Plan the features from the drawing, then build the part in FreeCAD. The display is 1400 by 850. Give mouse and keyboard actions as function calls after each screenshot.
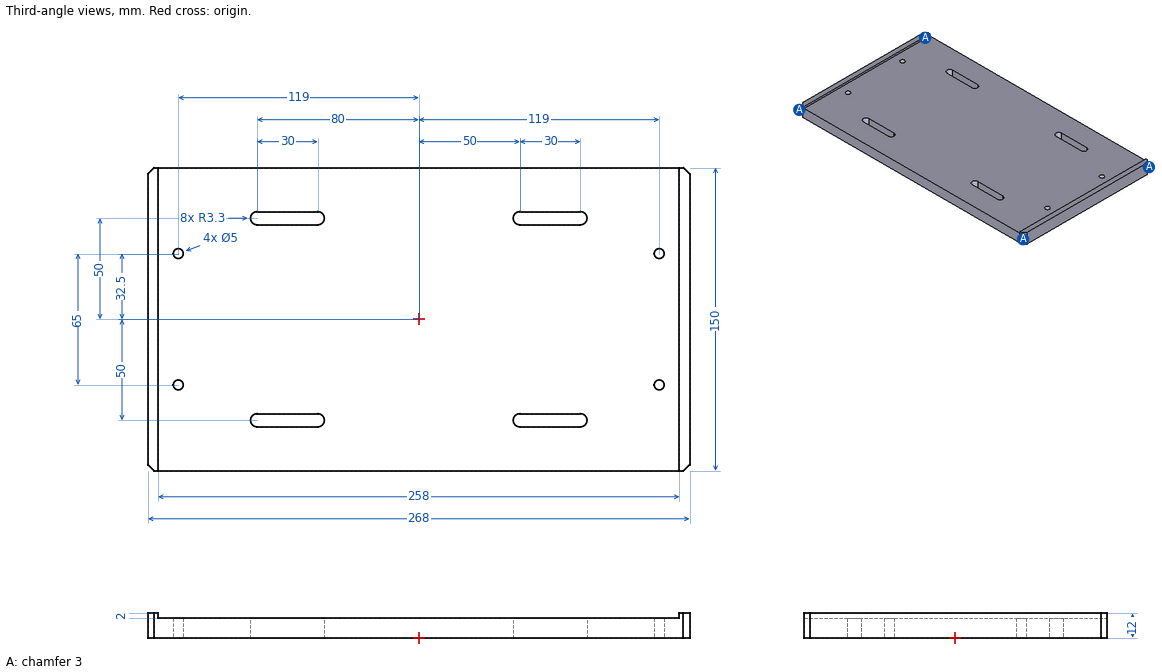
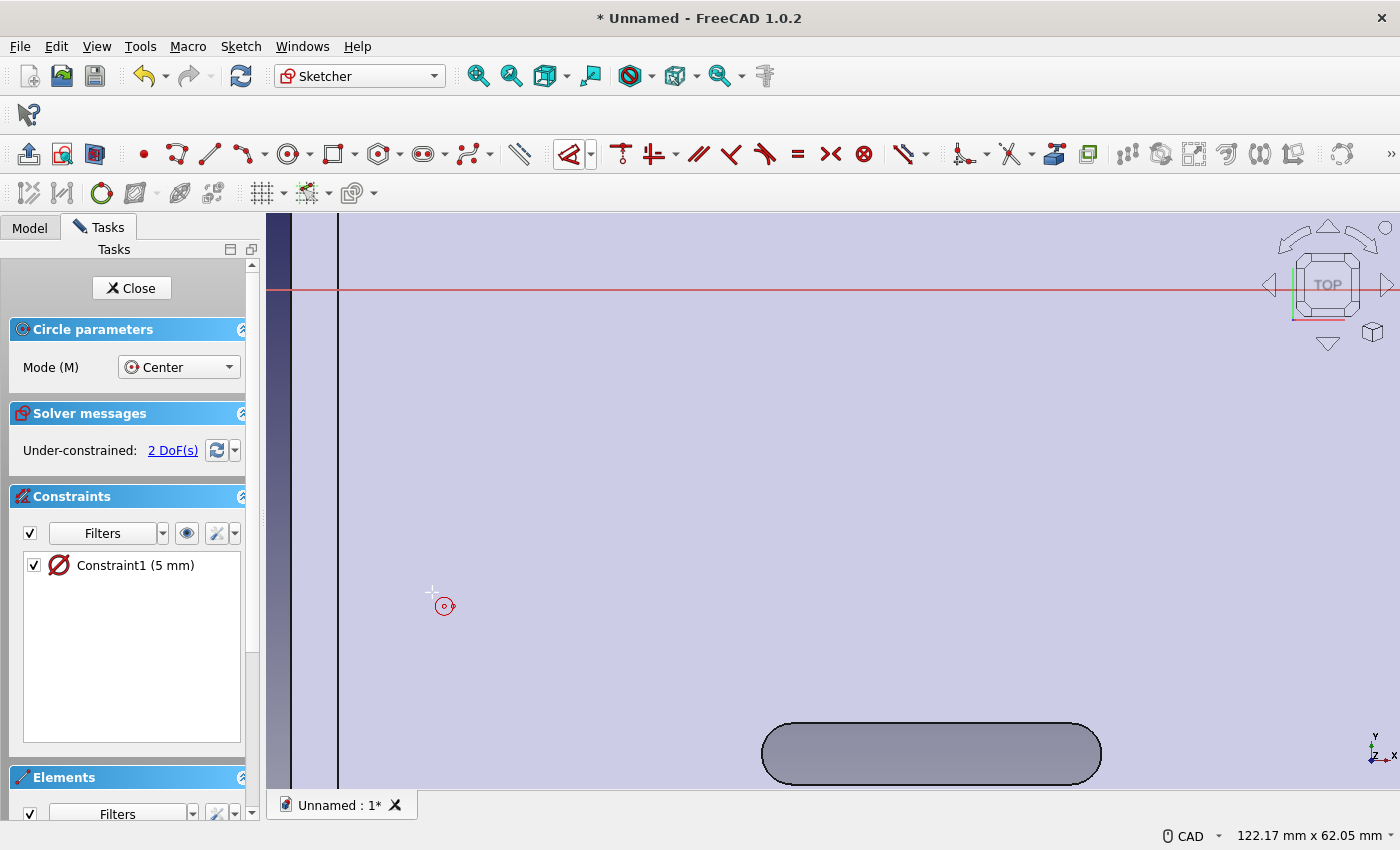
click(430, 592)
move(447, 575)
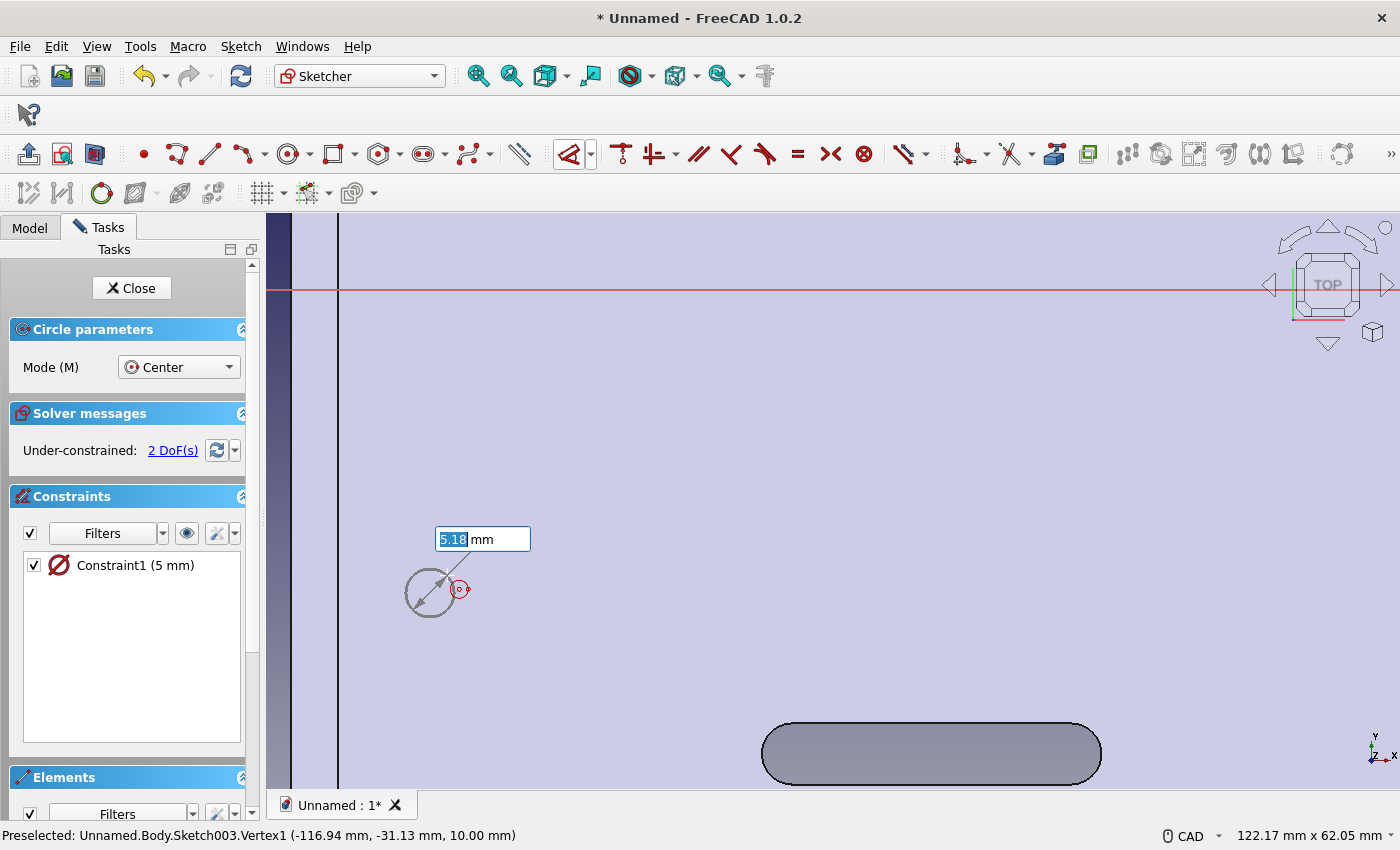
text(5)
key(Return)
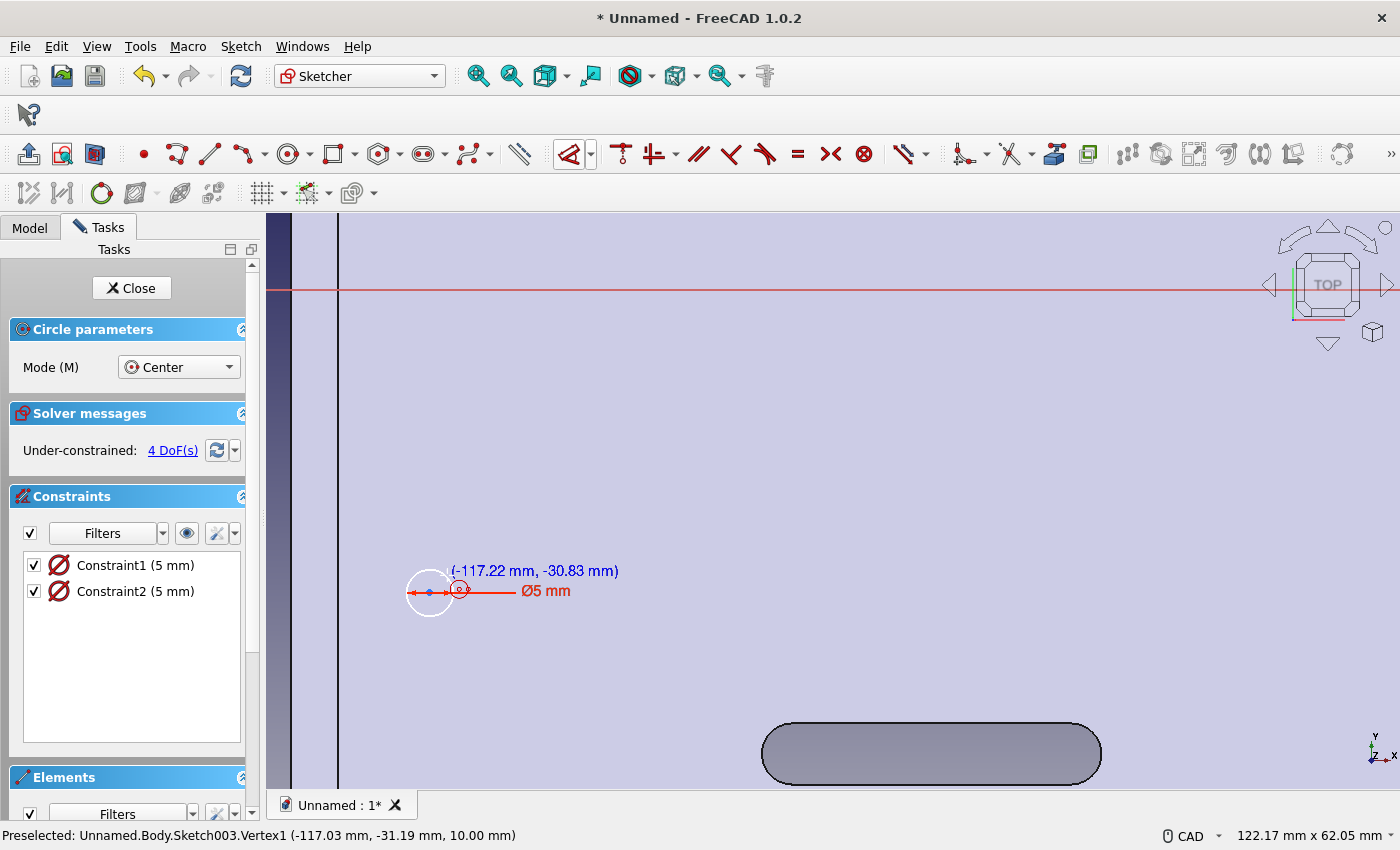
scroll(432, 592, down, 6)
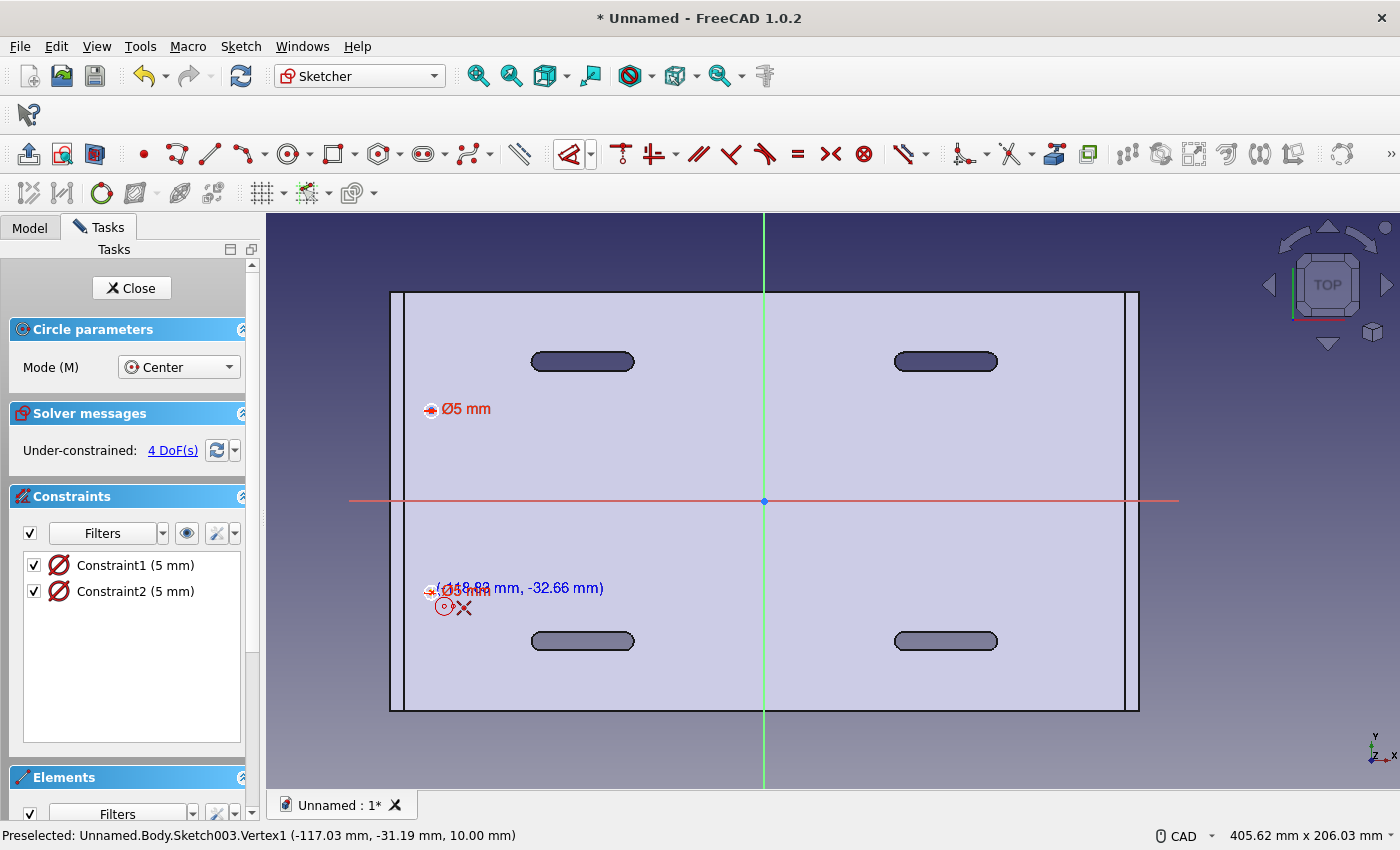
scroll(1097, 411, up, 6)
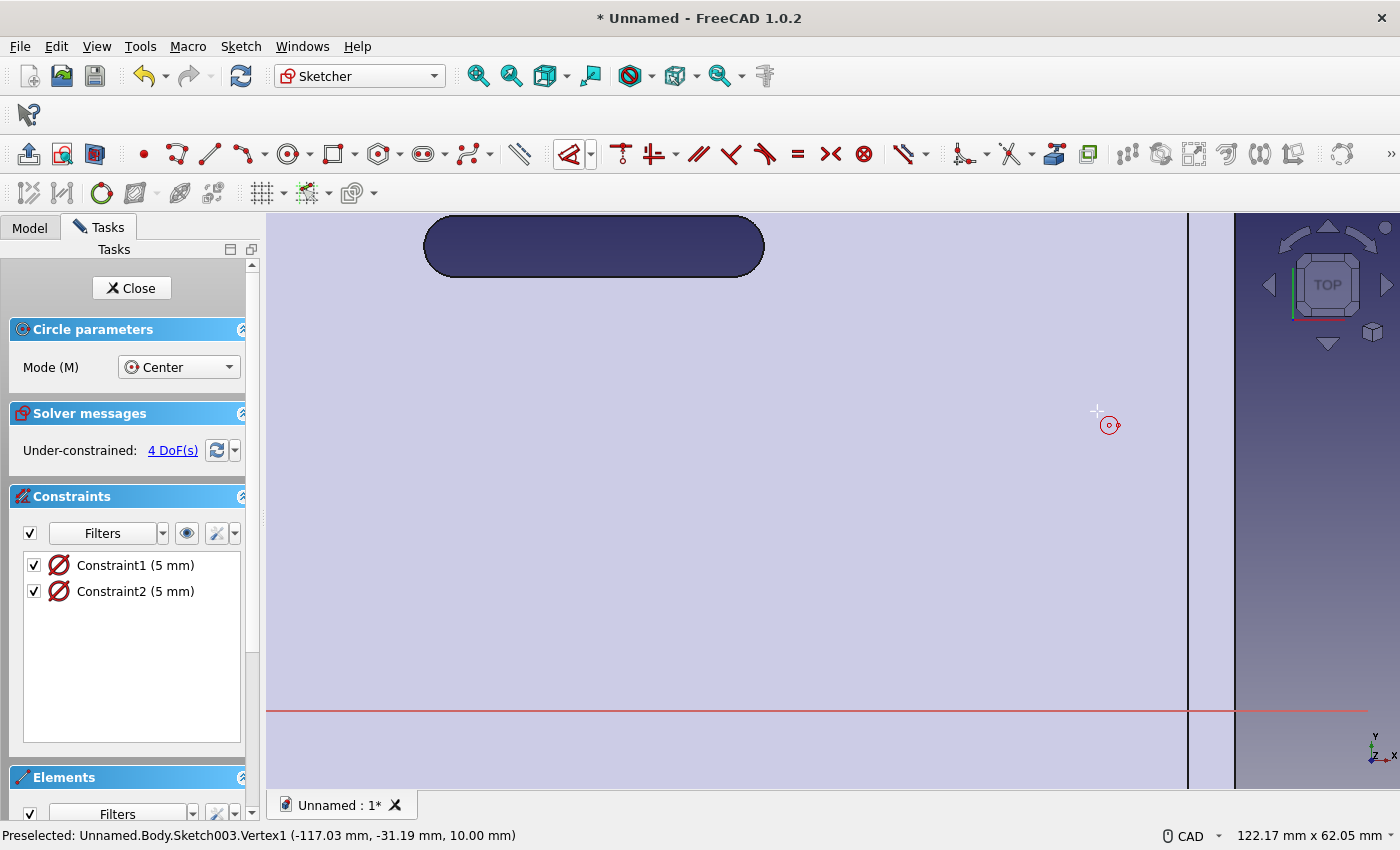
click(1095, 409)
move(1112, 392)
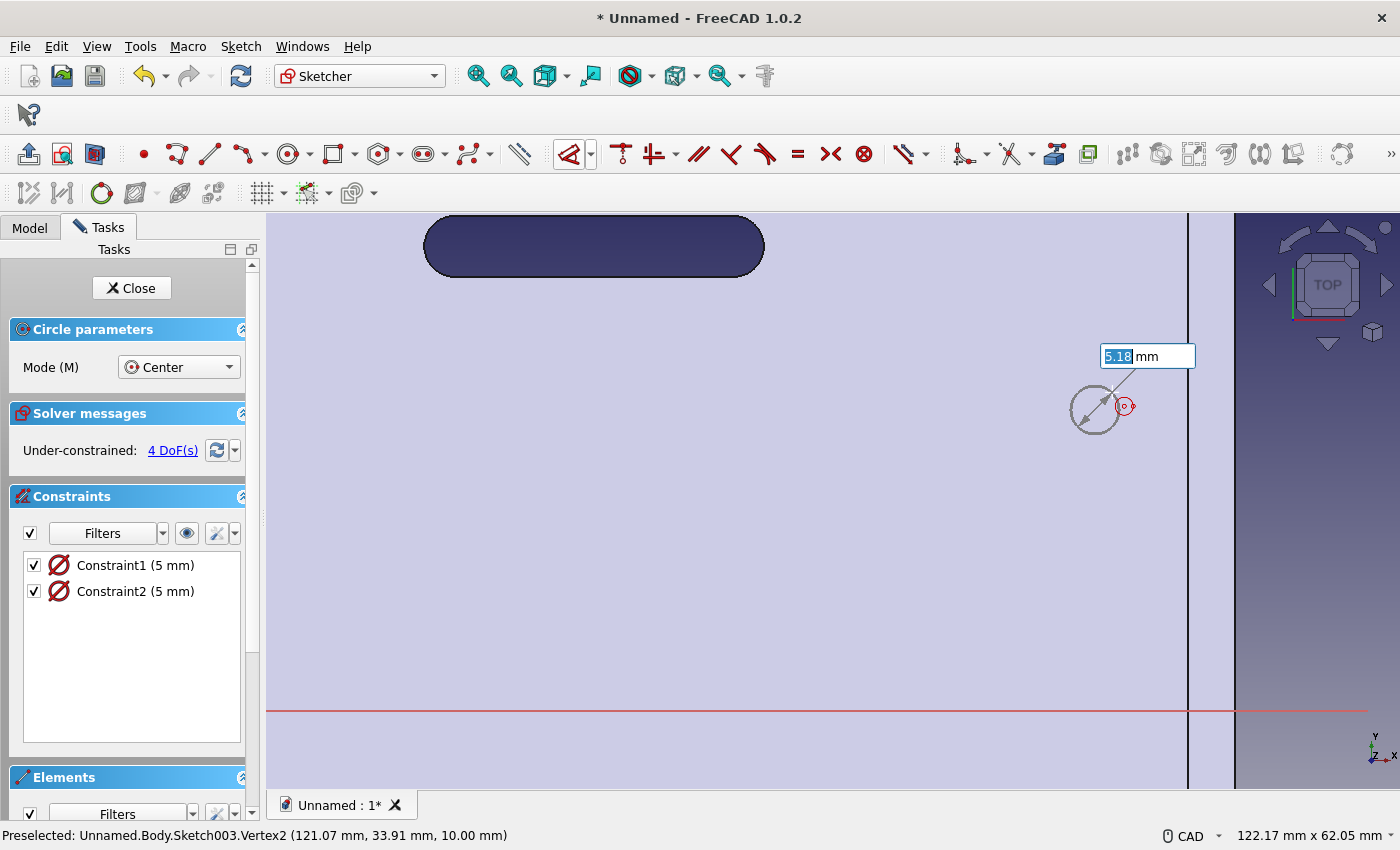
text(5)
key(Return)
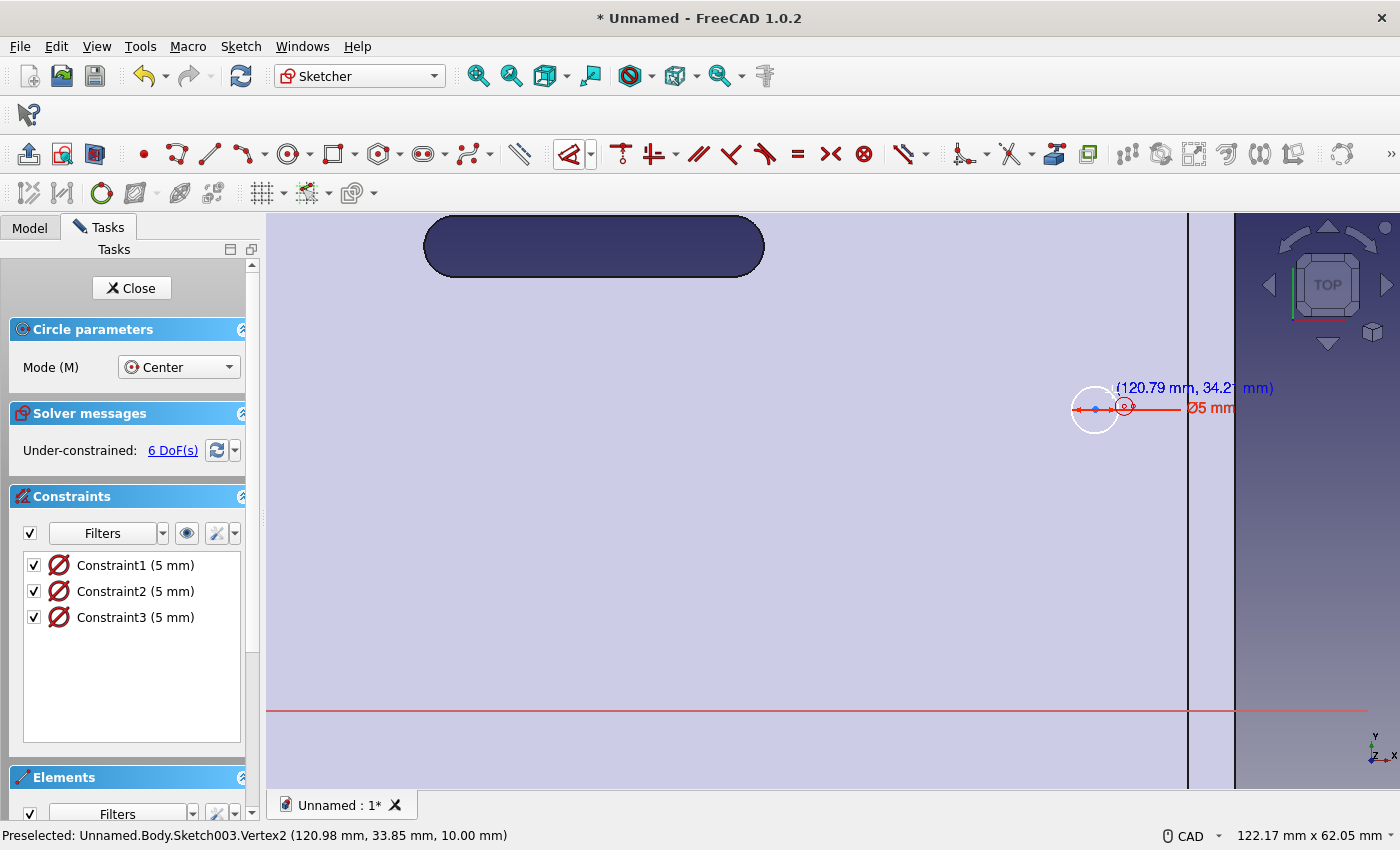
scroll(1098, 411, down, 6)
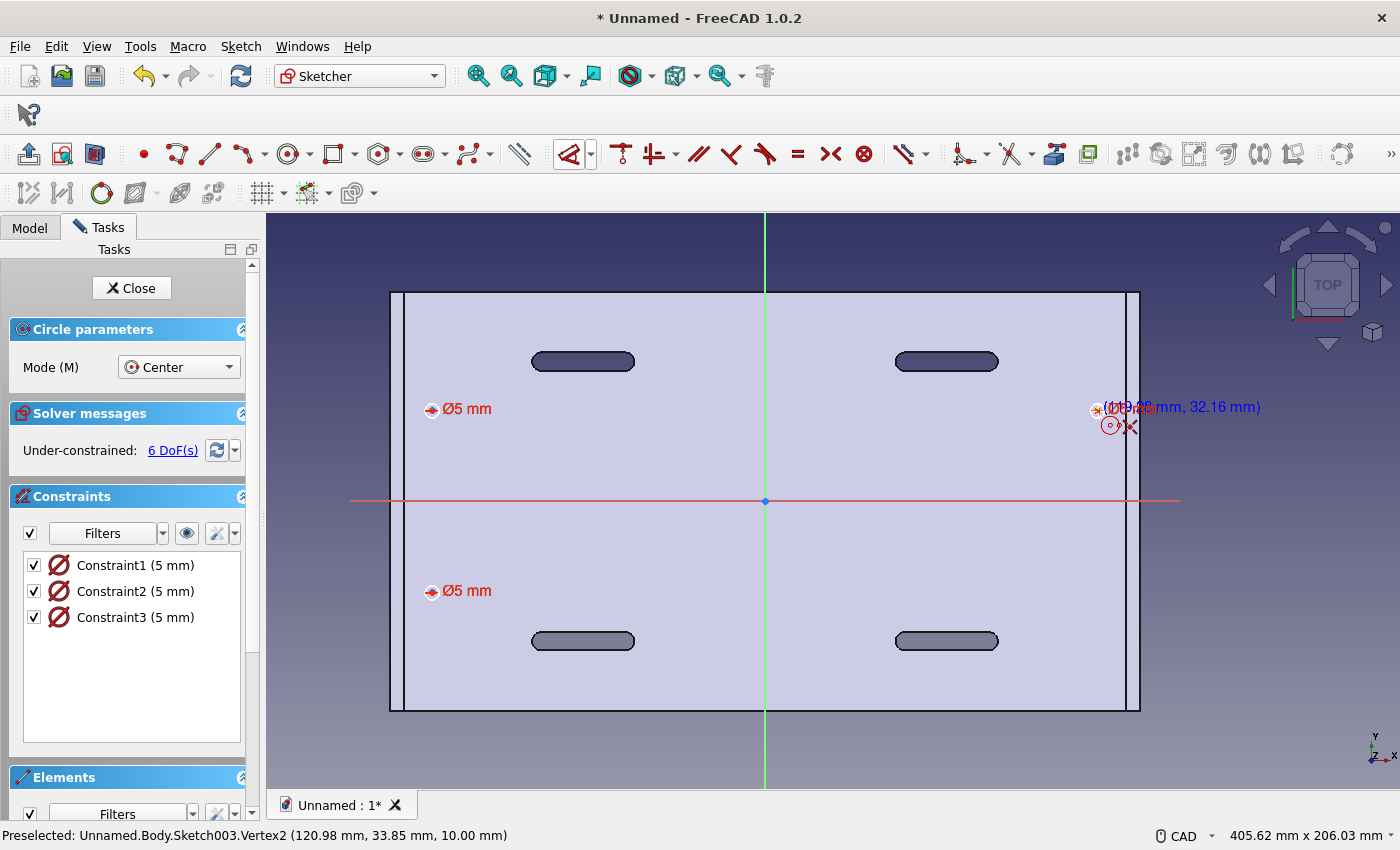
scroll(1098, 592, up, 6)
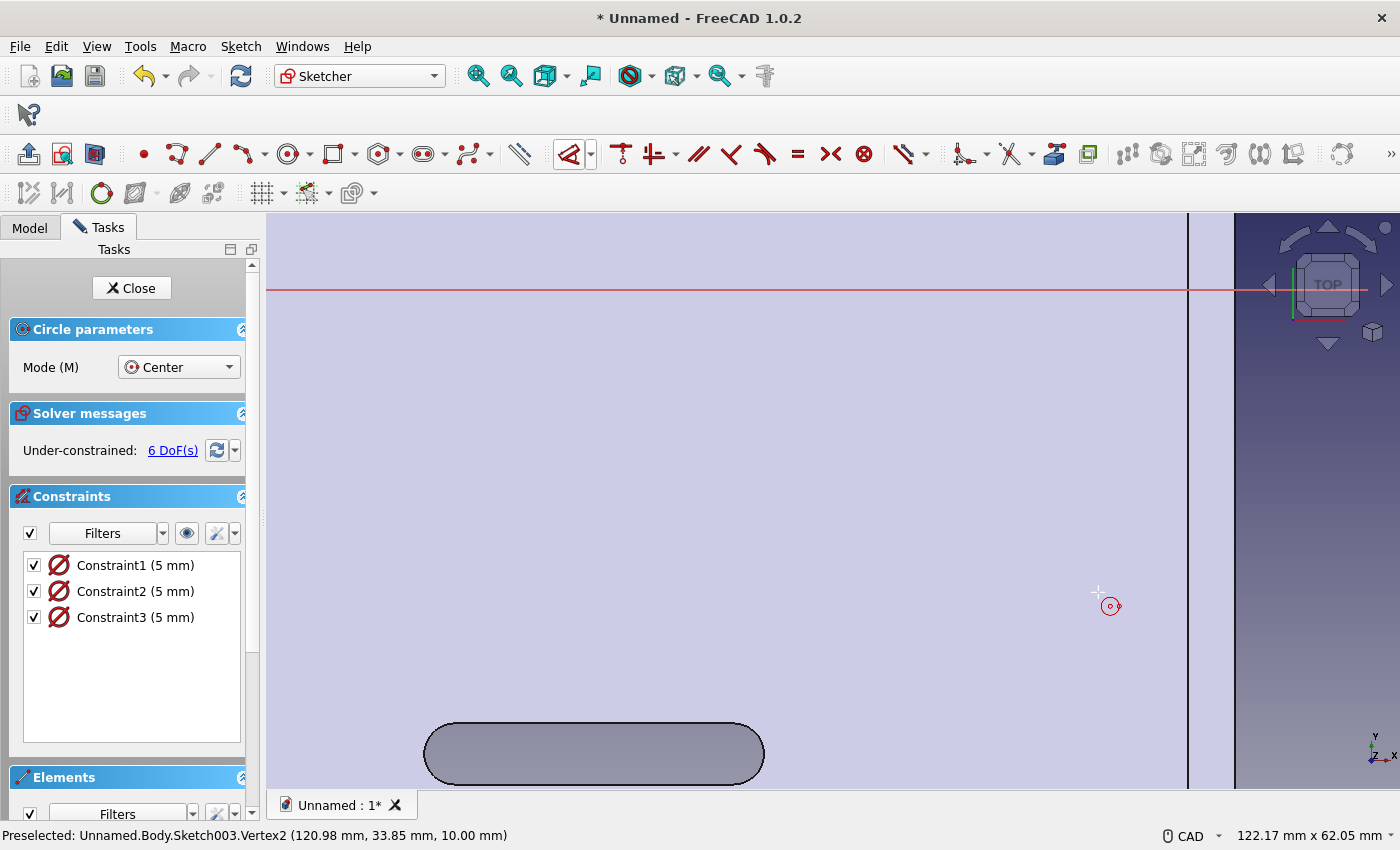
click(1095, 592)
move(1112, 575)